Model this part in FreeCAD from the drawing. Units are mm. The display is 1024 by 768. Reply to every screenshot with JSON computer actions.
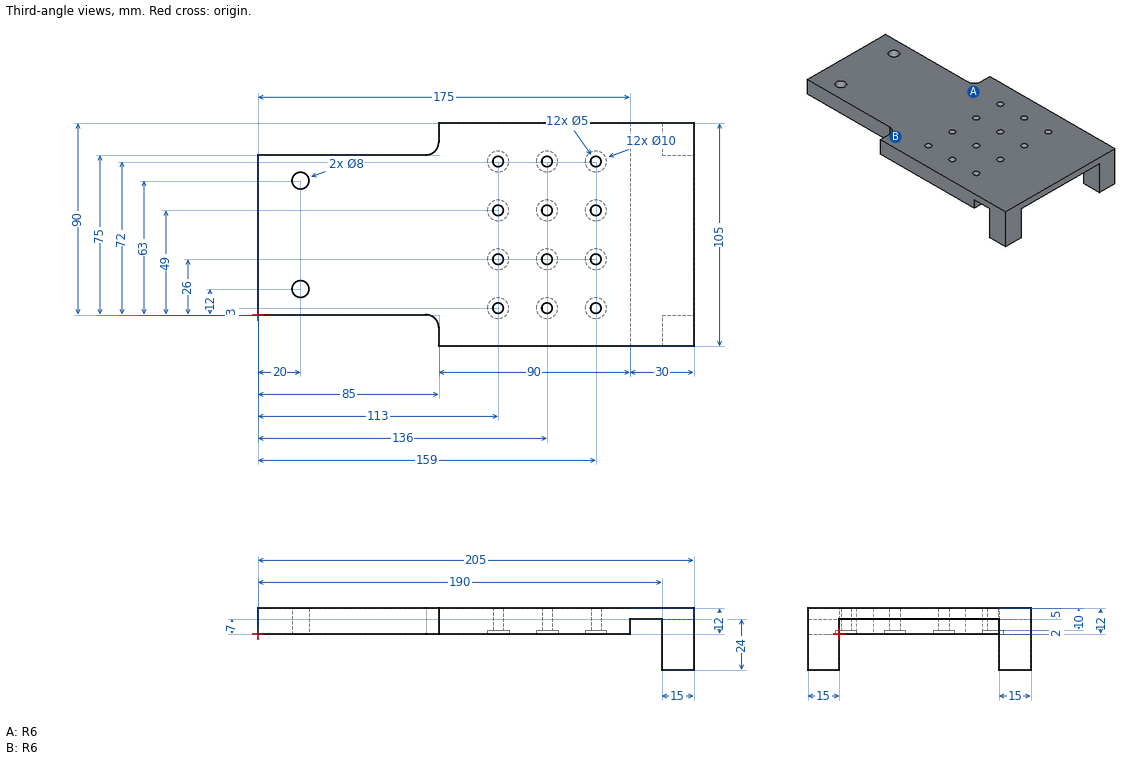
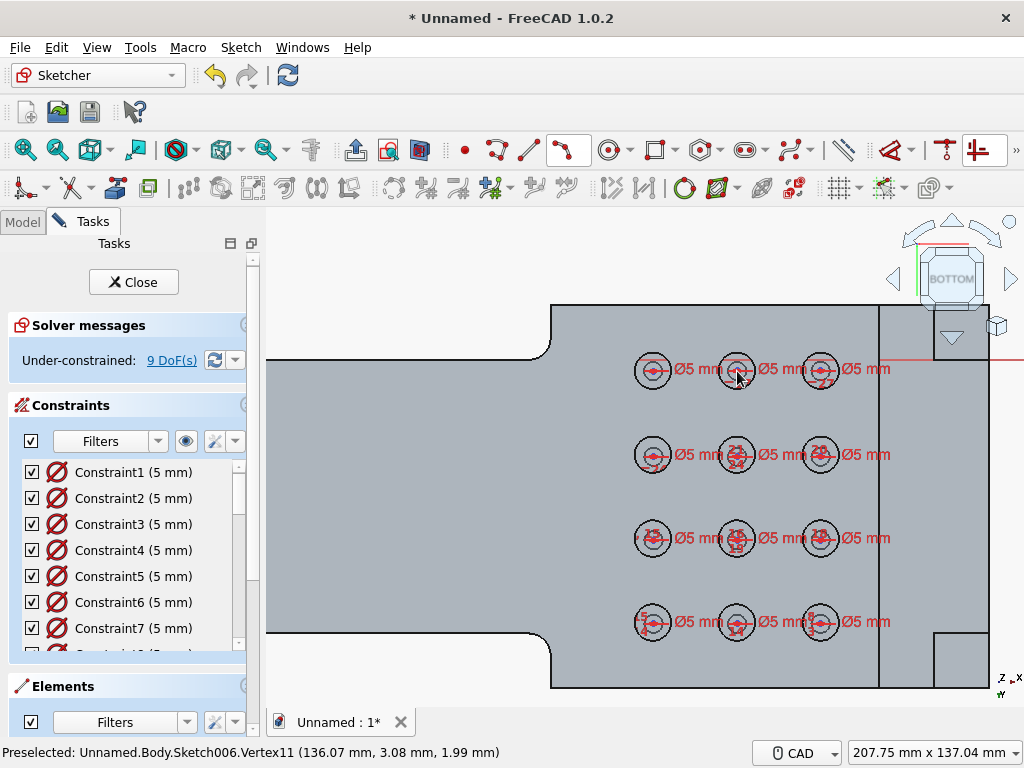
{"action": "left_click", "coordinate": [654, 457]}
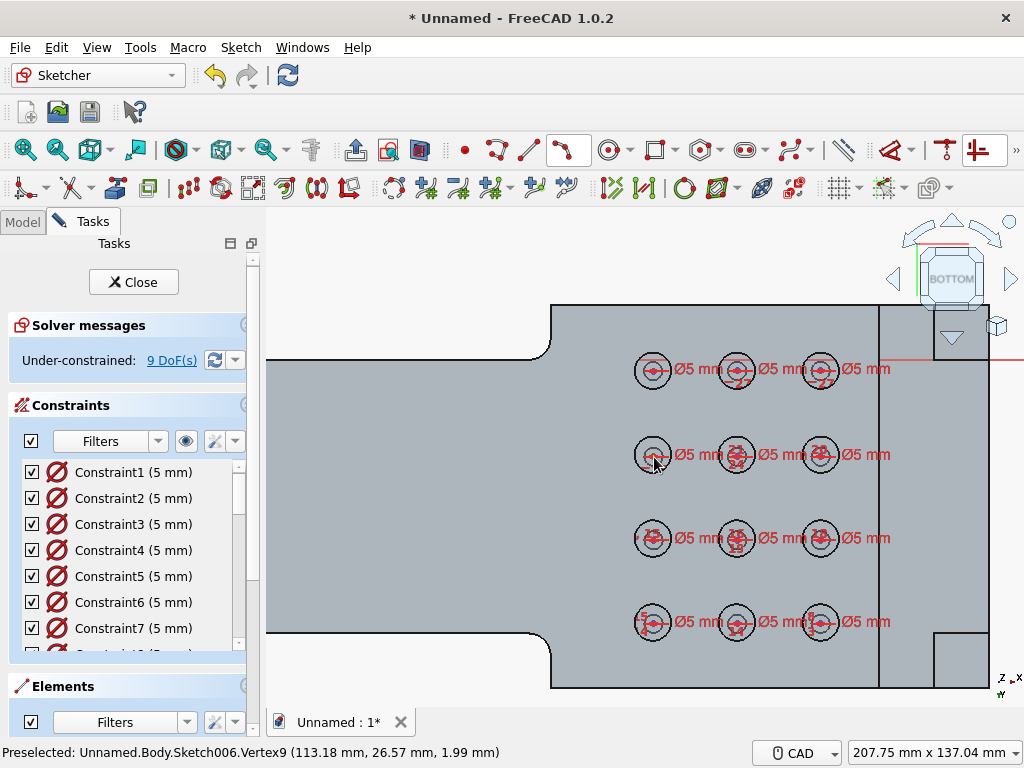
{"action": "left_click", "coordinate": [653, 371]}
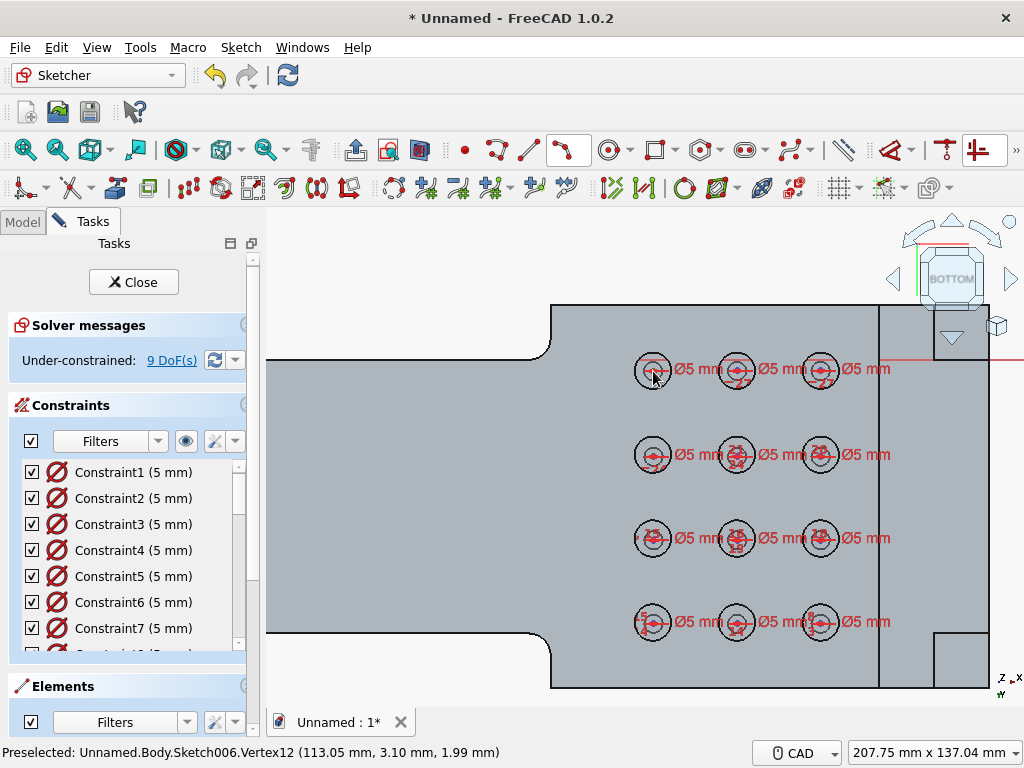
{"action": "key", "text": "v"}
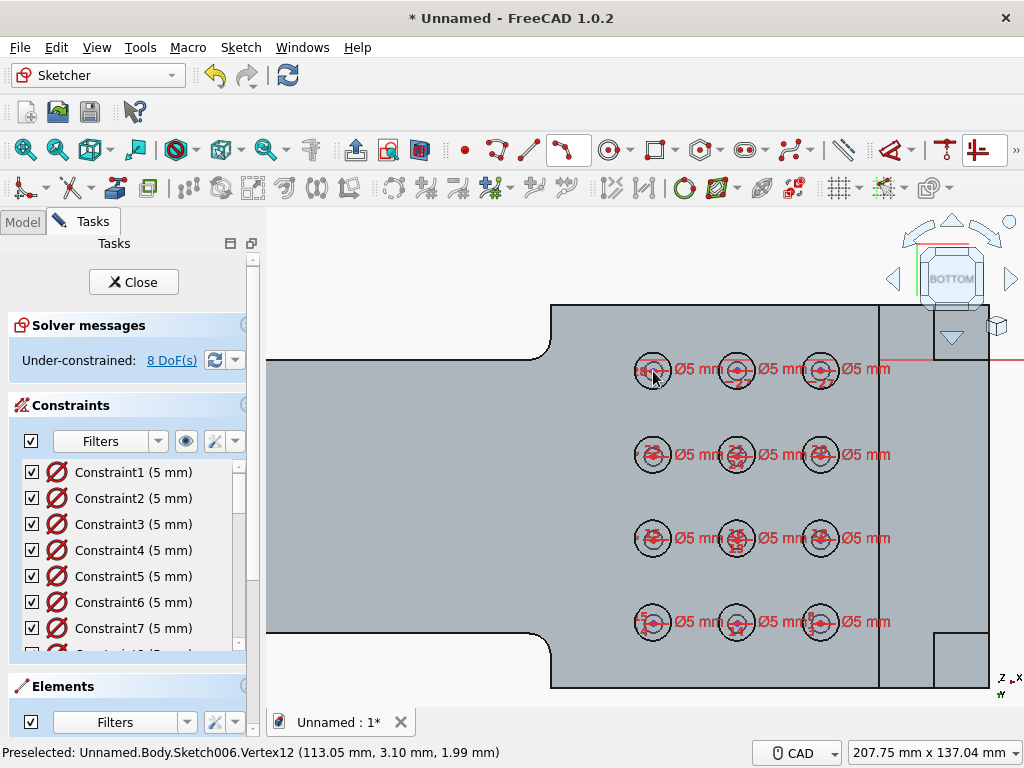
{"action": "left_click", "coordinate": [737, 371]}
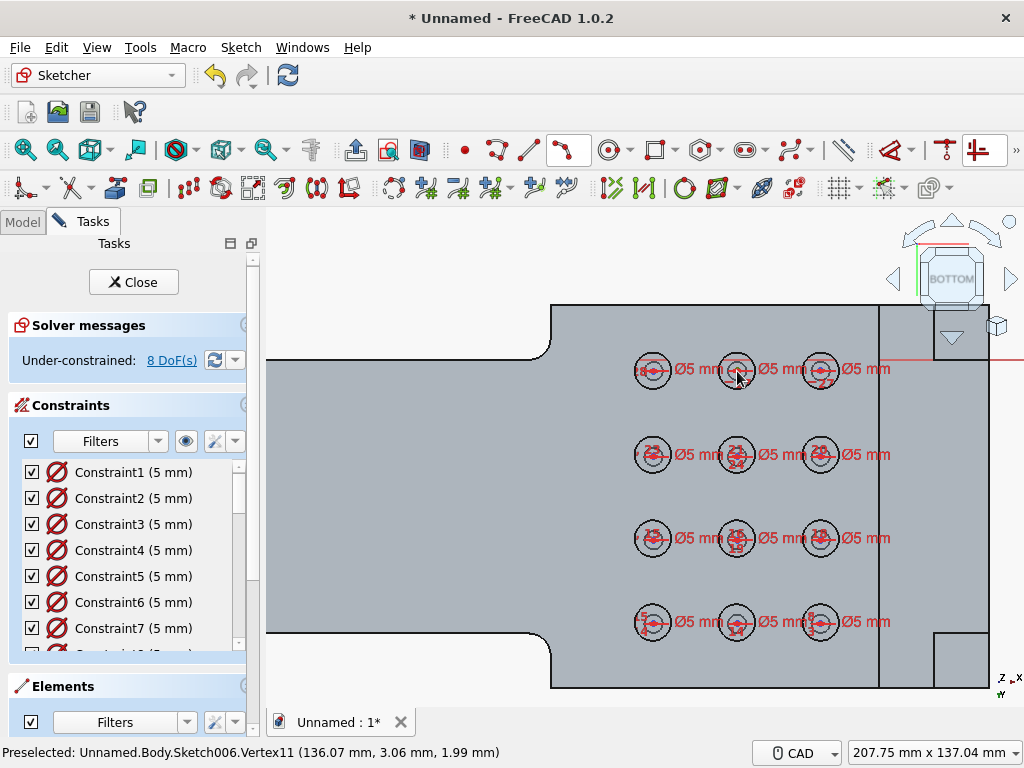
{"action": "left_click", "coordinate": [654, 371]}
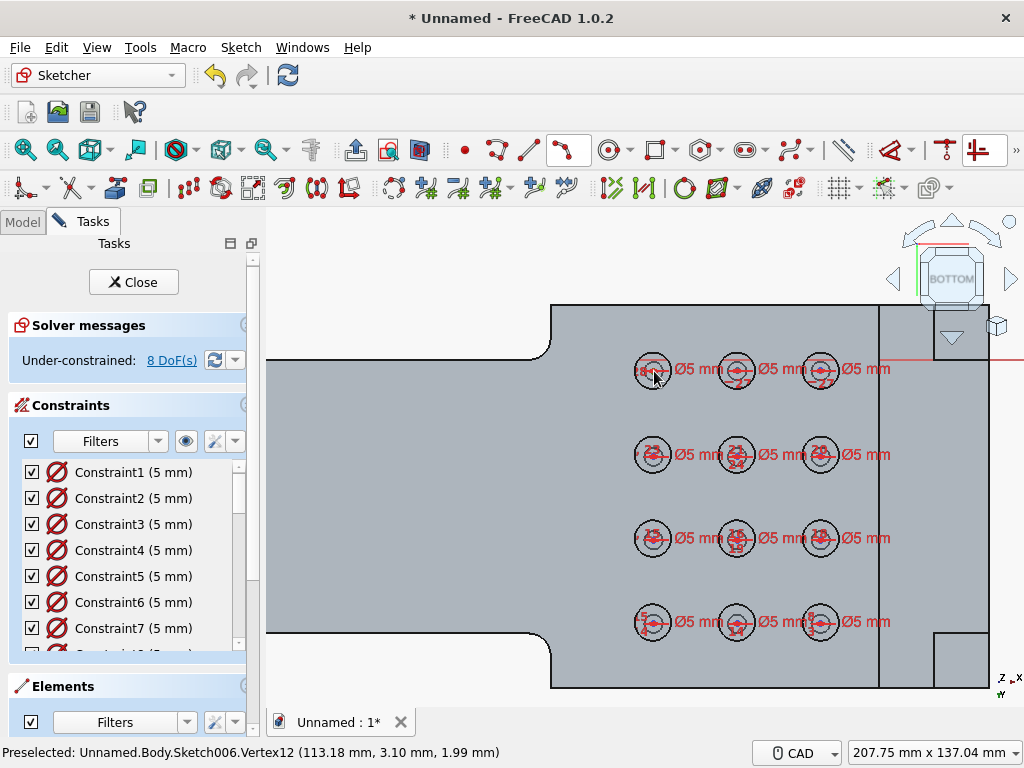
{"action": "key", "text": "h"}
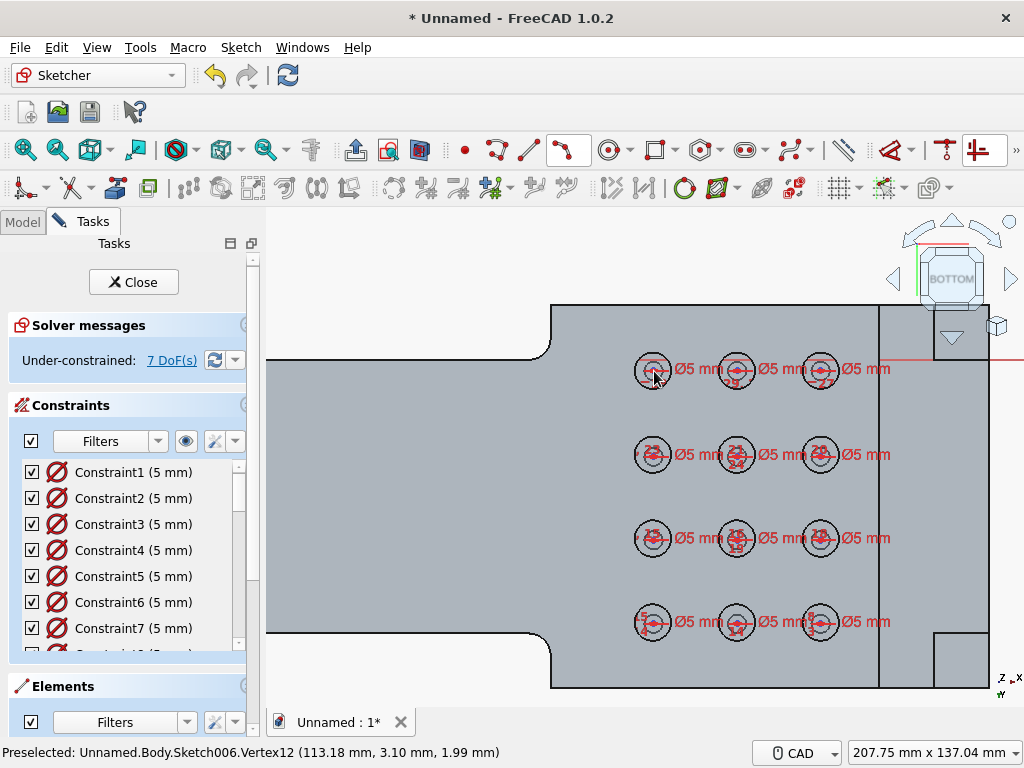
{"action": "left_click", "coordinate": [890, 150]}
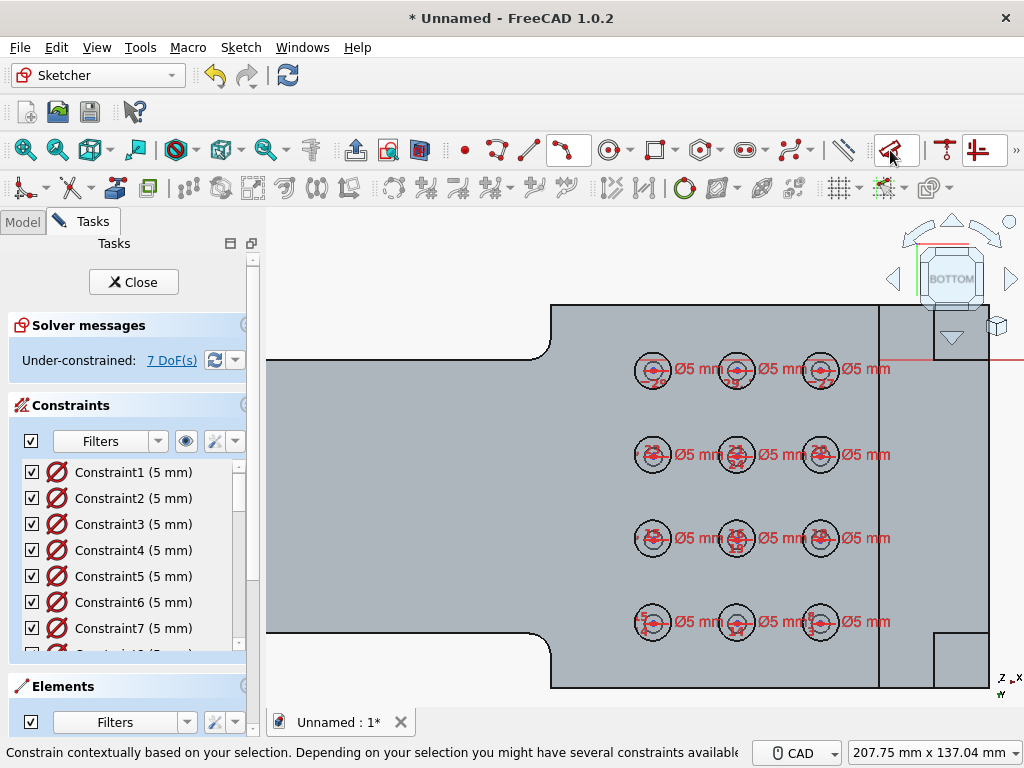
{"action": "scroll", "coordinate": [821, 371], "scroll_direction": "up", "scroll_amount": 7}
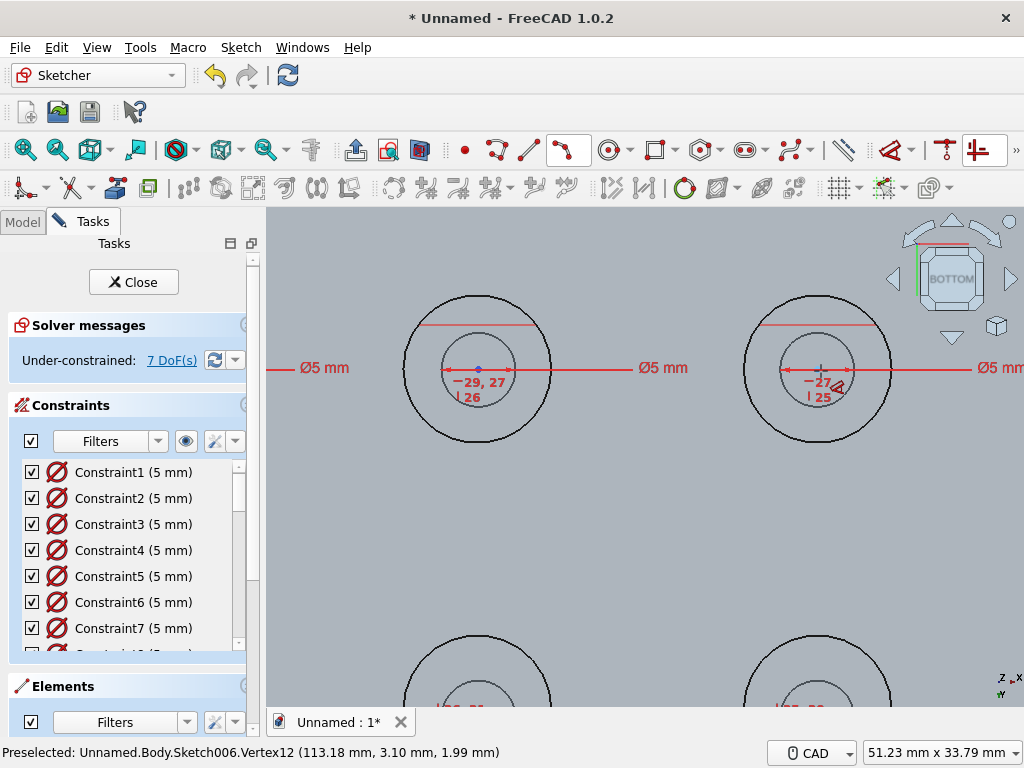
{"action": "left_click", "coordinate": [817, 370]}
{"action": "left_click", "coordinate": [851, 337]}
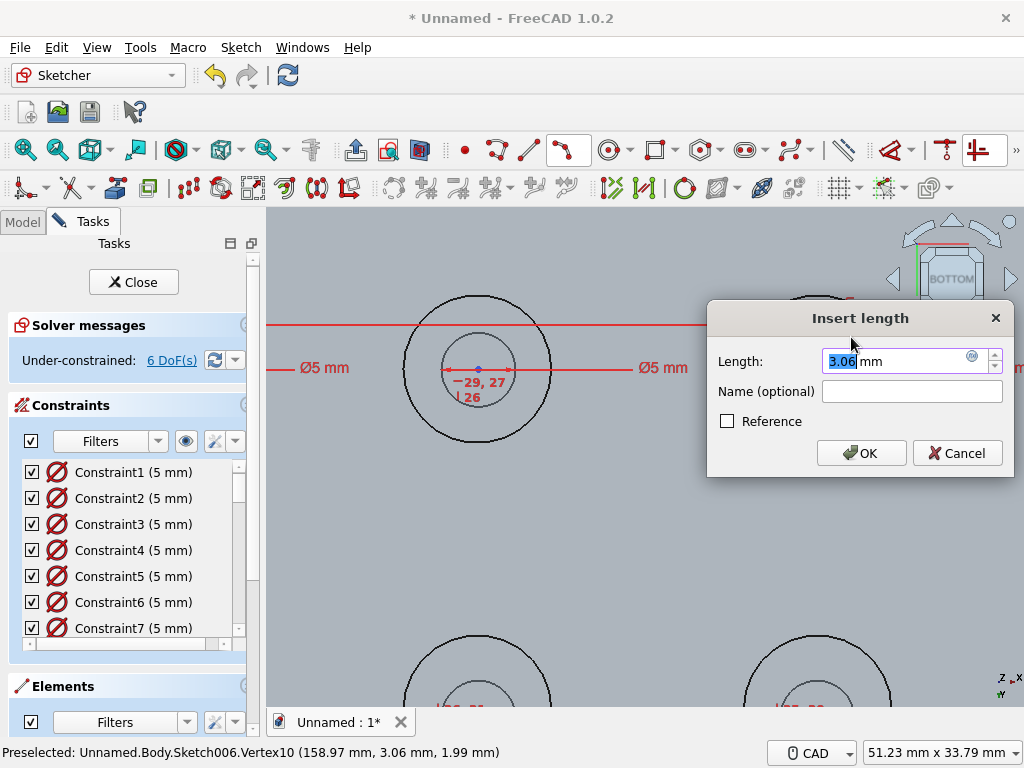
{"action": "type", "text": "3"}
{"action": "key", "text": "Return"}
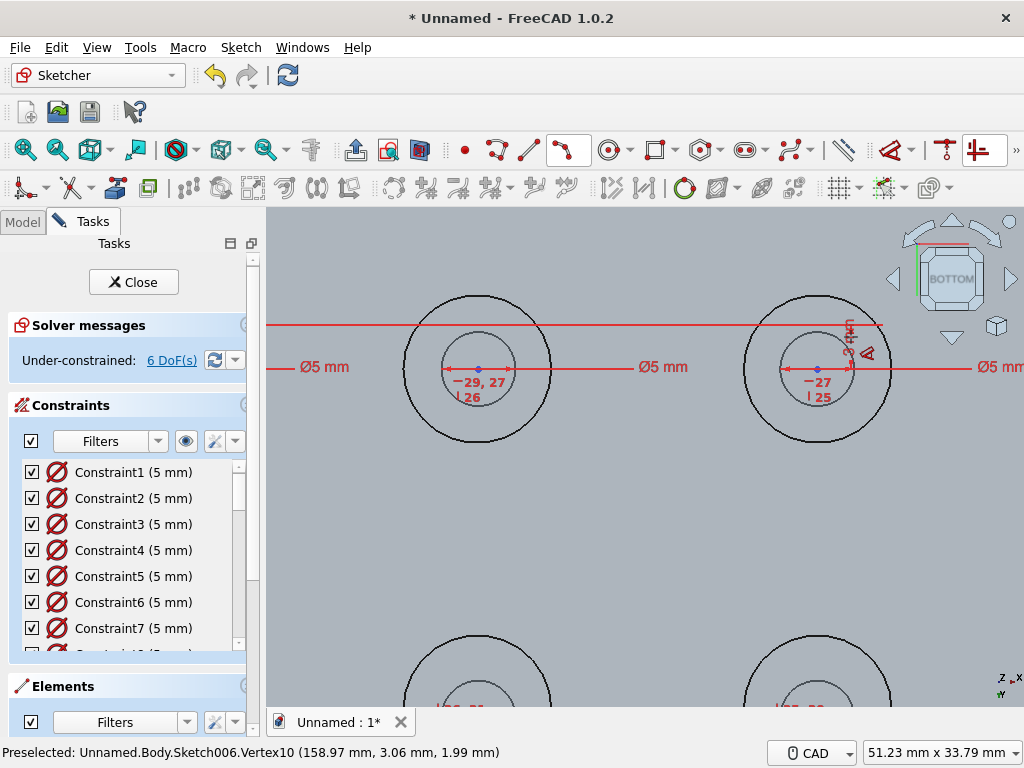
{"action": "scroll", "coordinate": [758, 374], "scroll_direction": "down", "scroll_amount": 9}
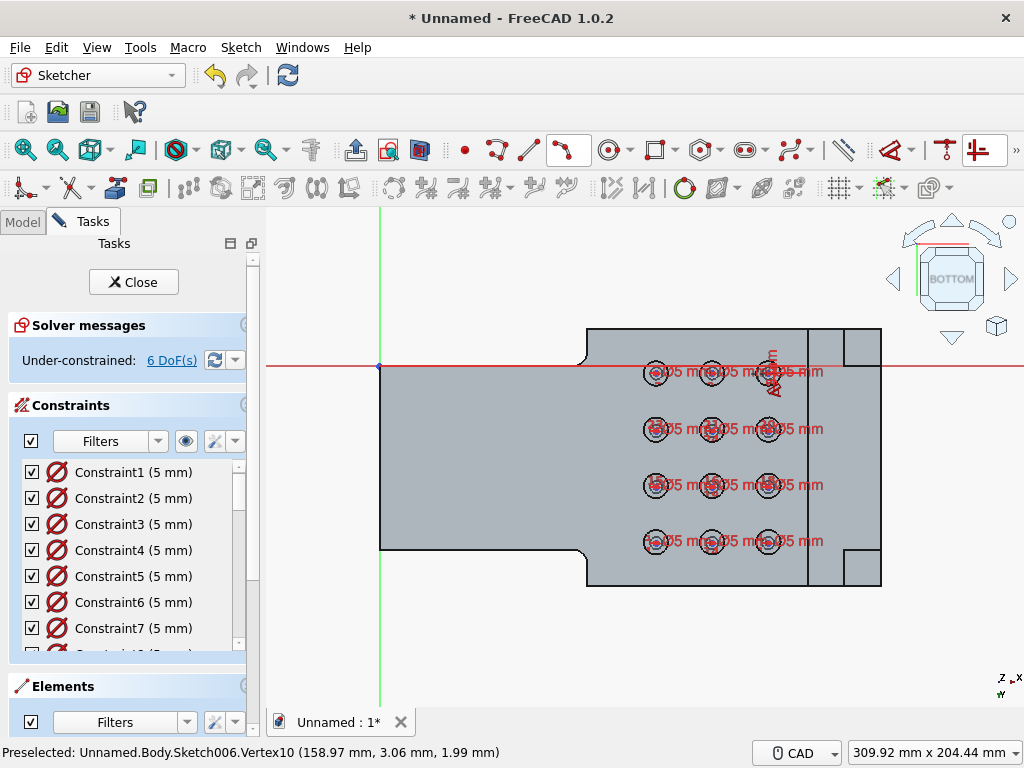
{"action": "left_click", "coordinate": [768, 543]}
{"action": "left_click", "coordinate": [346, 455]}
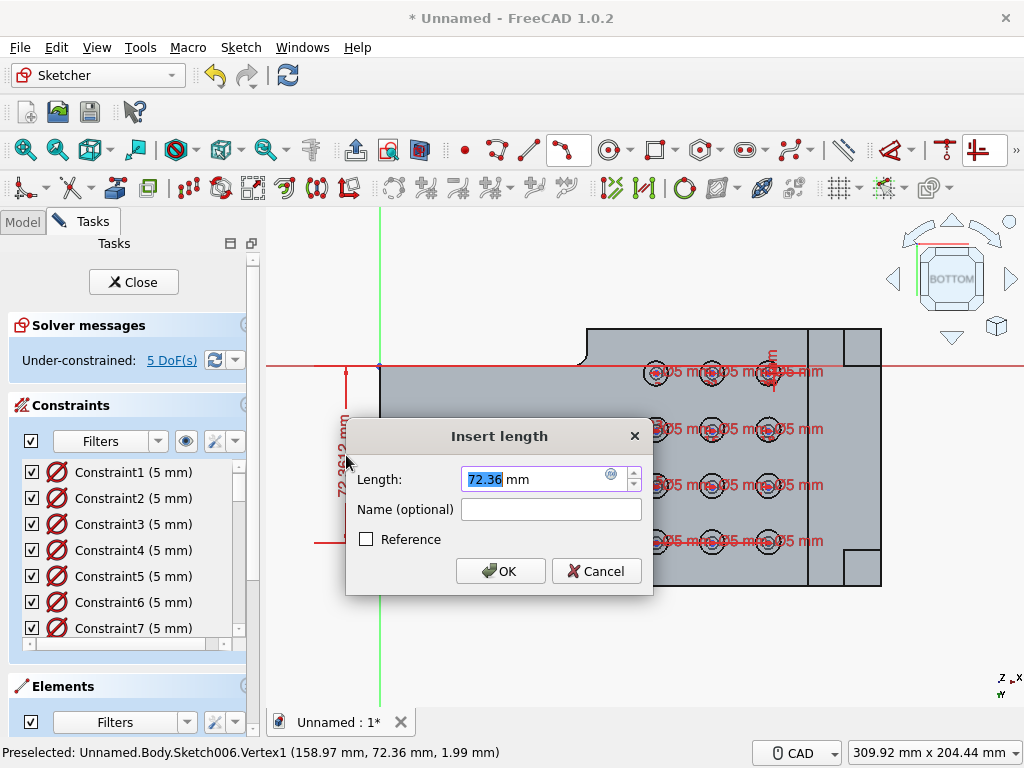
{"action": "type", "text": "72"}
{"action": "key", "text": "Return"}